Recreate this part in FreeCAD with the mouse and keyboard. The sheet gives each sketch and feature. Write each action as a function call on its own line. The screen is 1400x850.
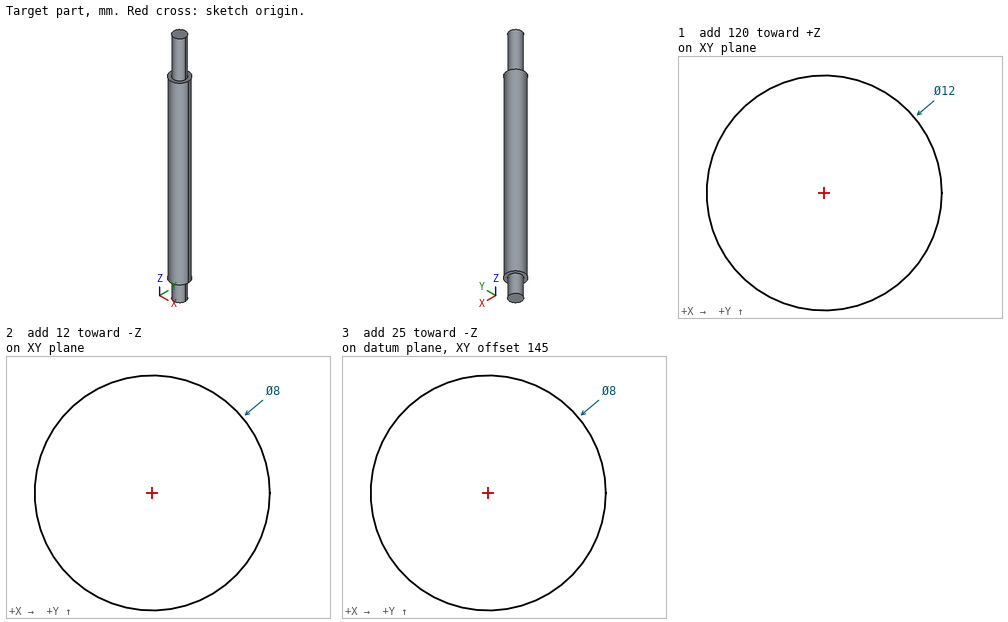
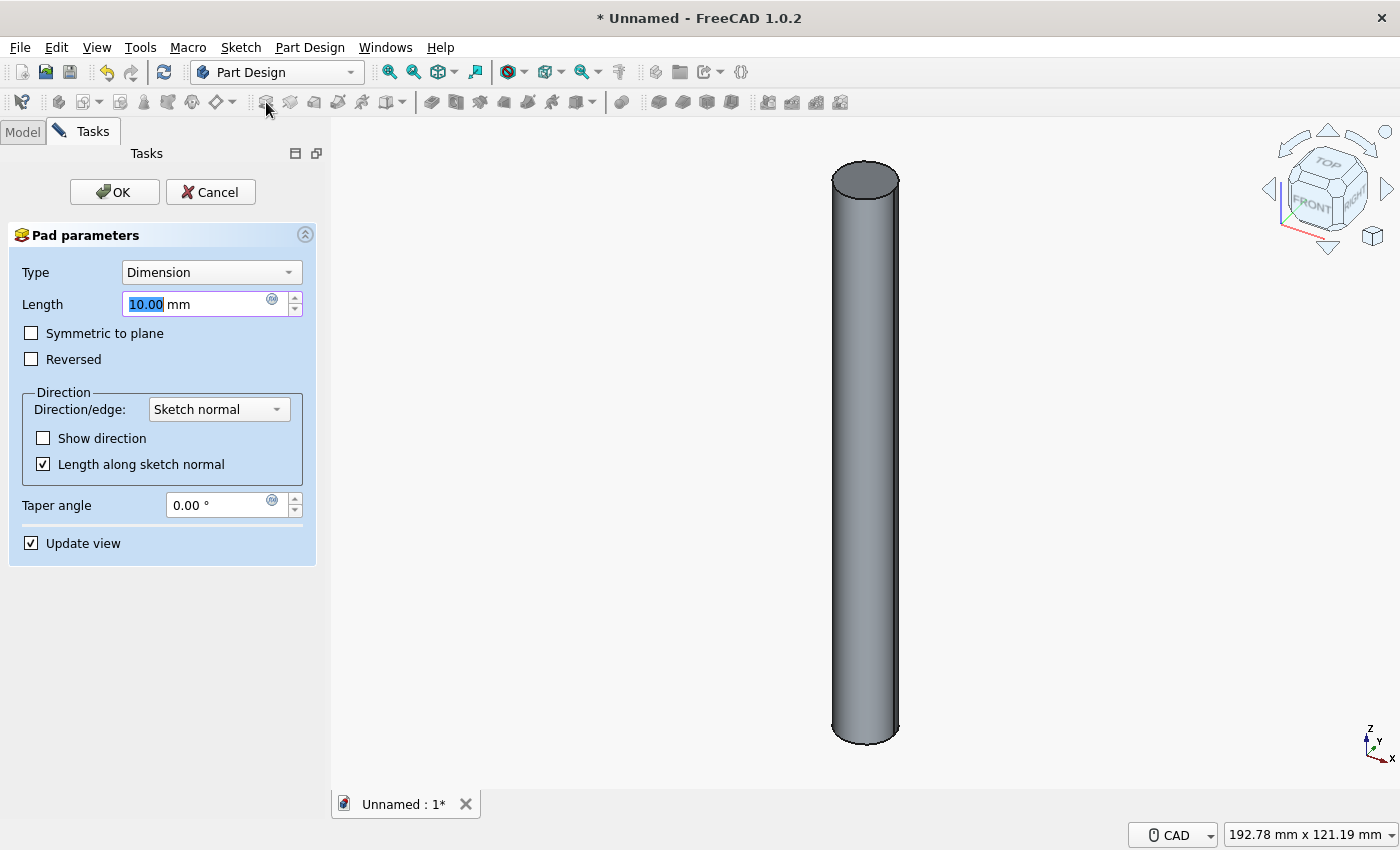
text(12)
key(Tab)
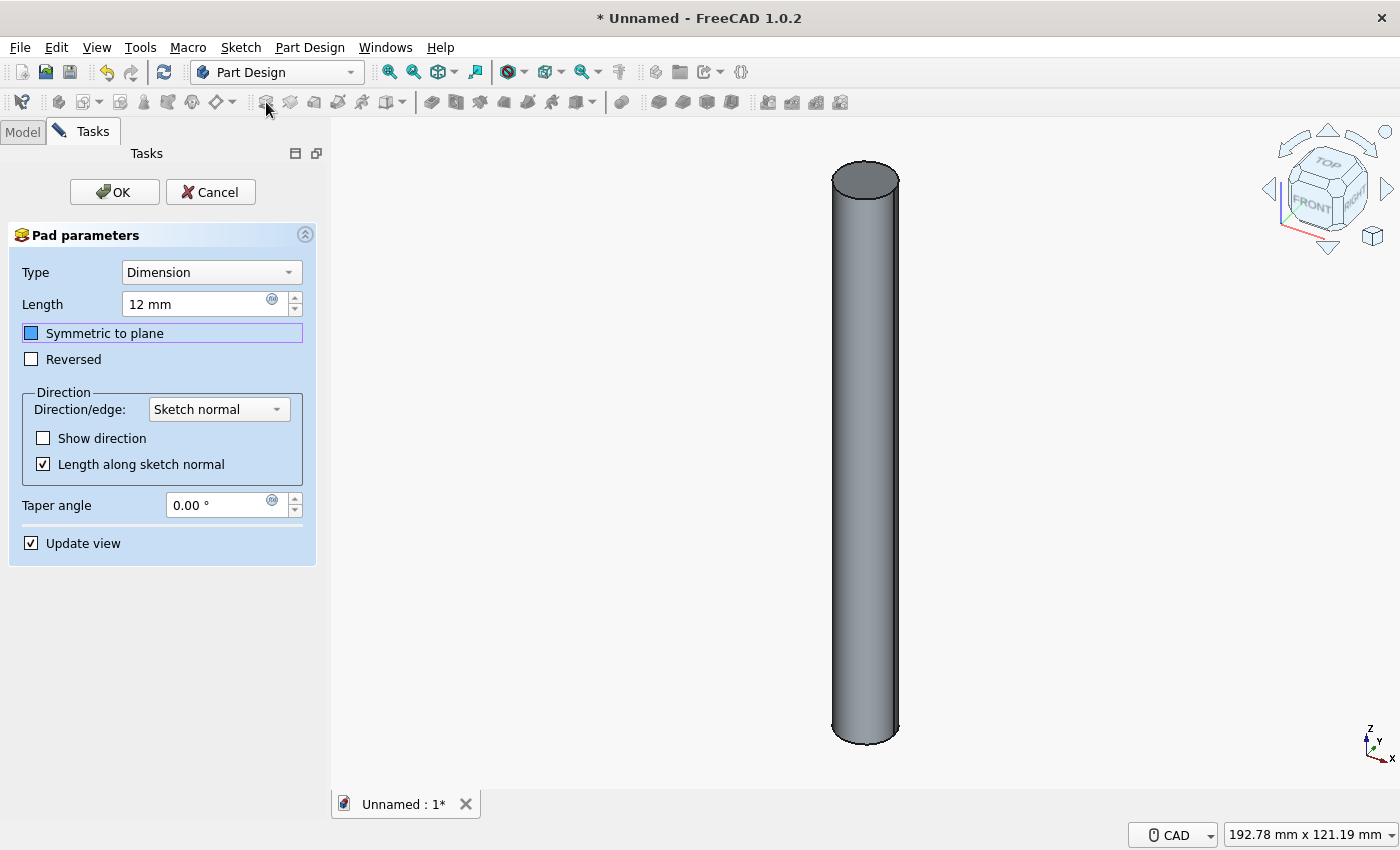
click(30, 359)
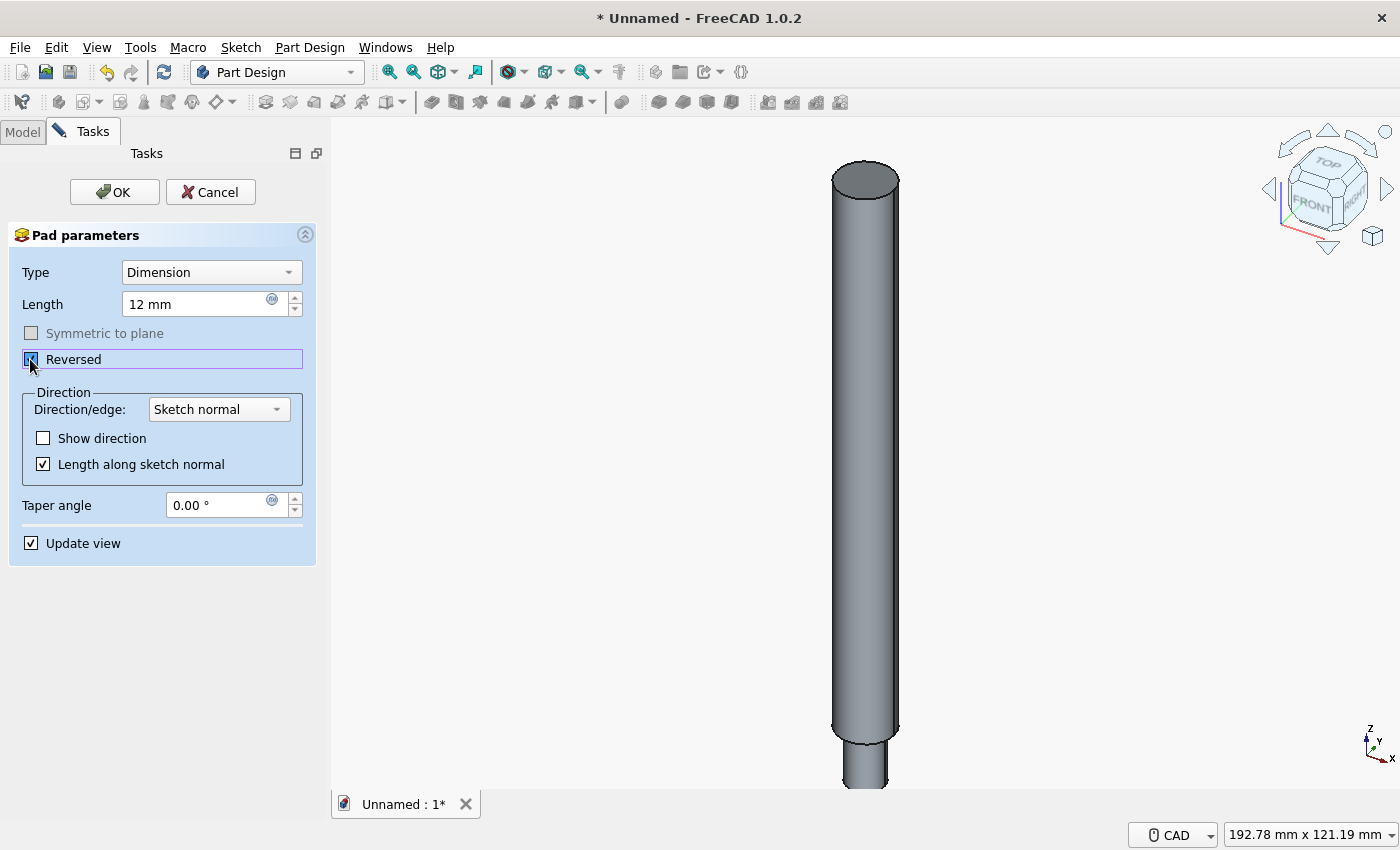
click(115, 192)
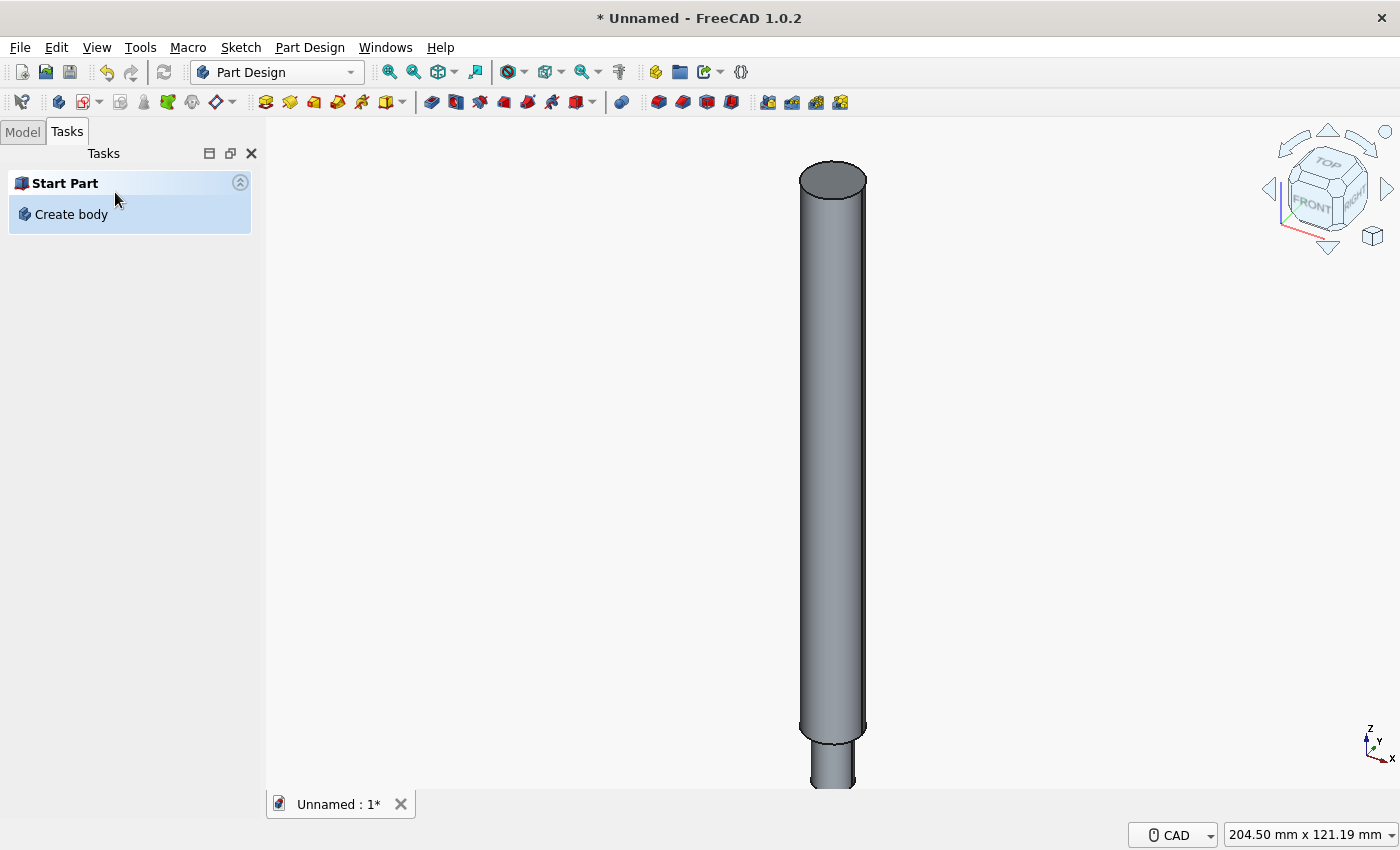
key(v)
key(f)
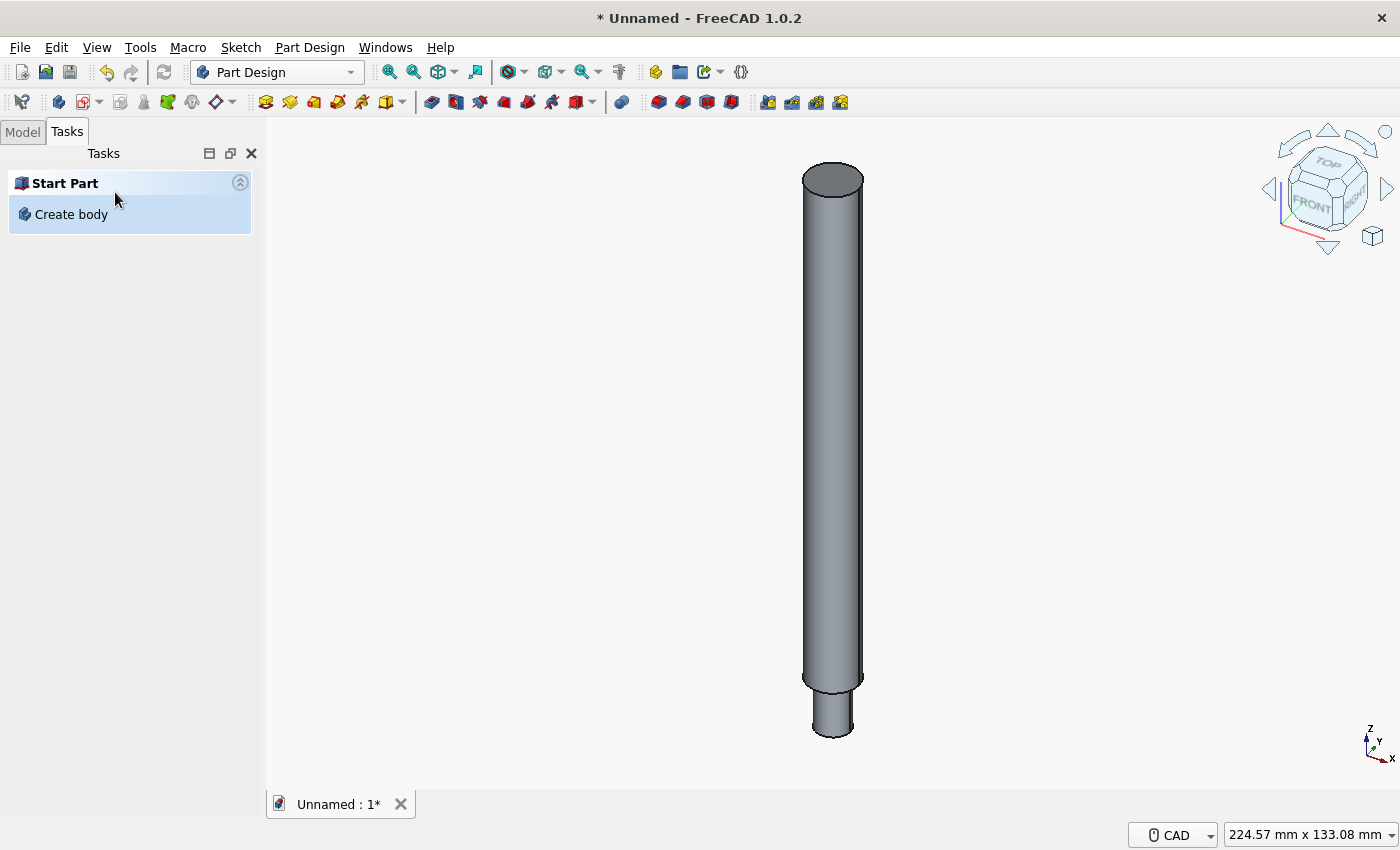
click(23, 131)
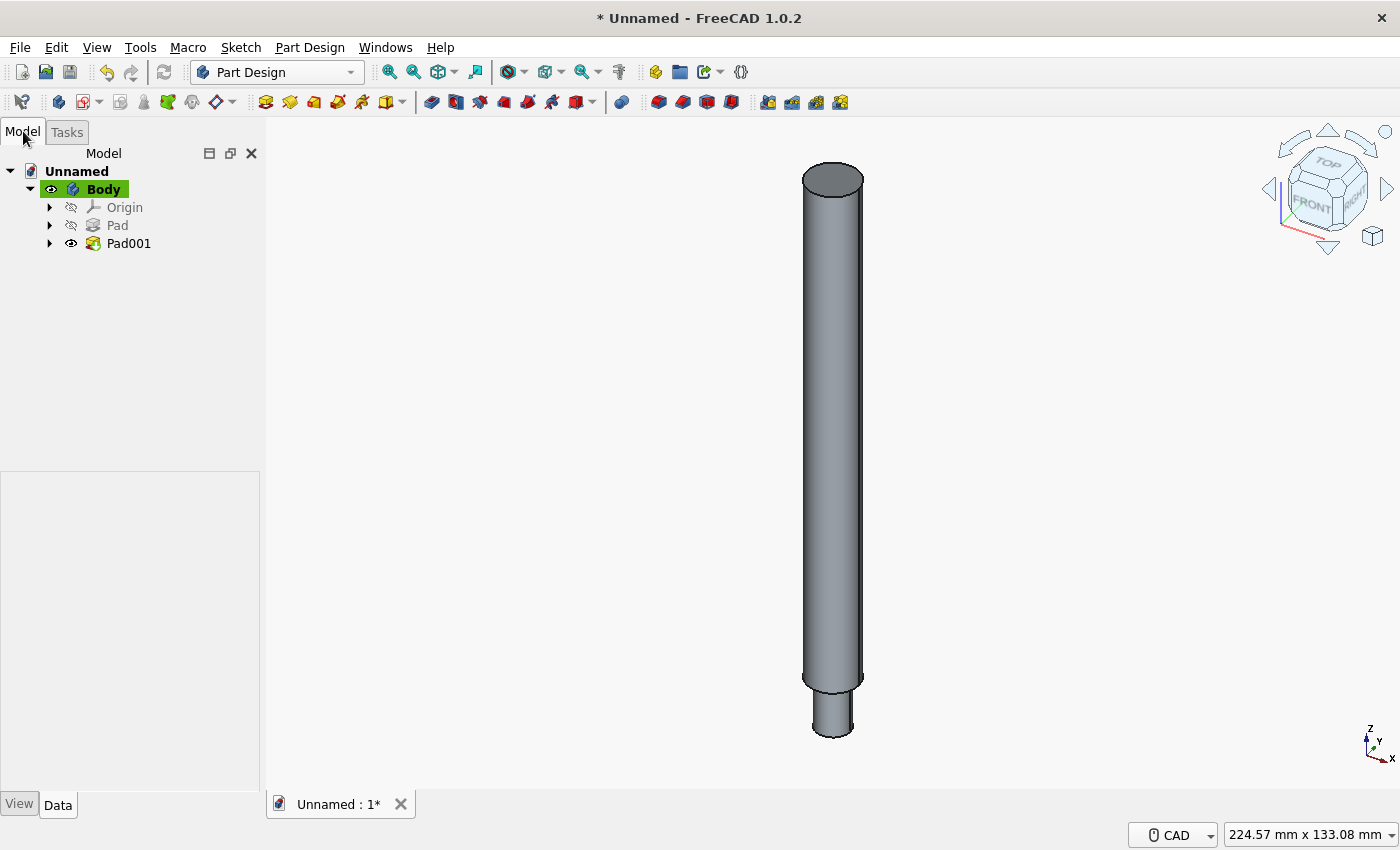
click(50, 207)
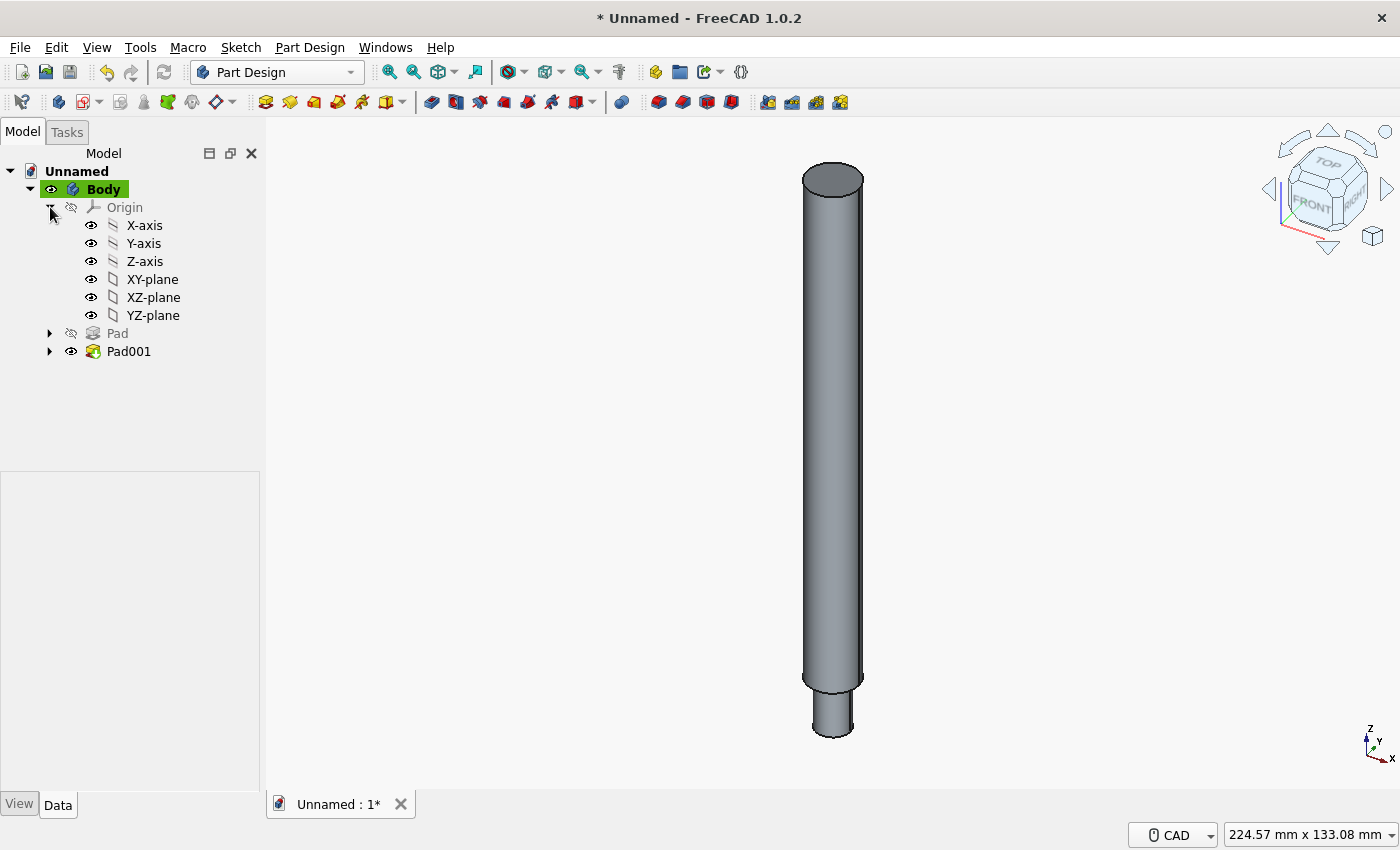
click(136, 279)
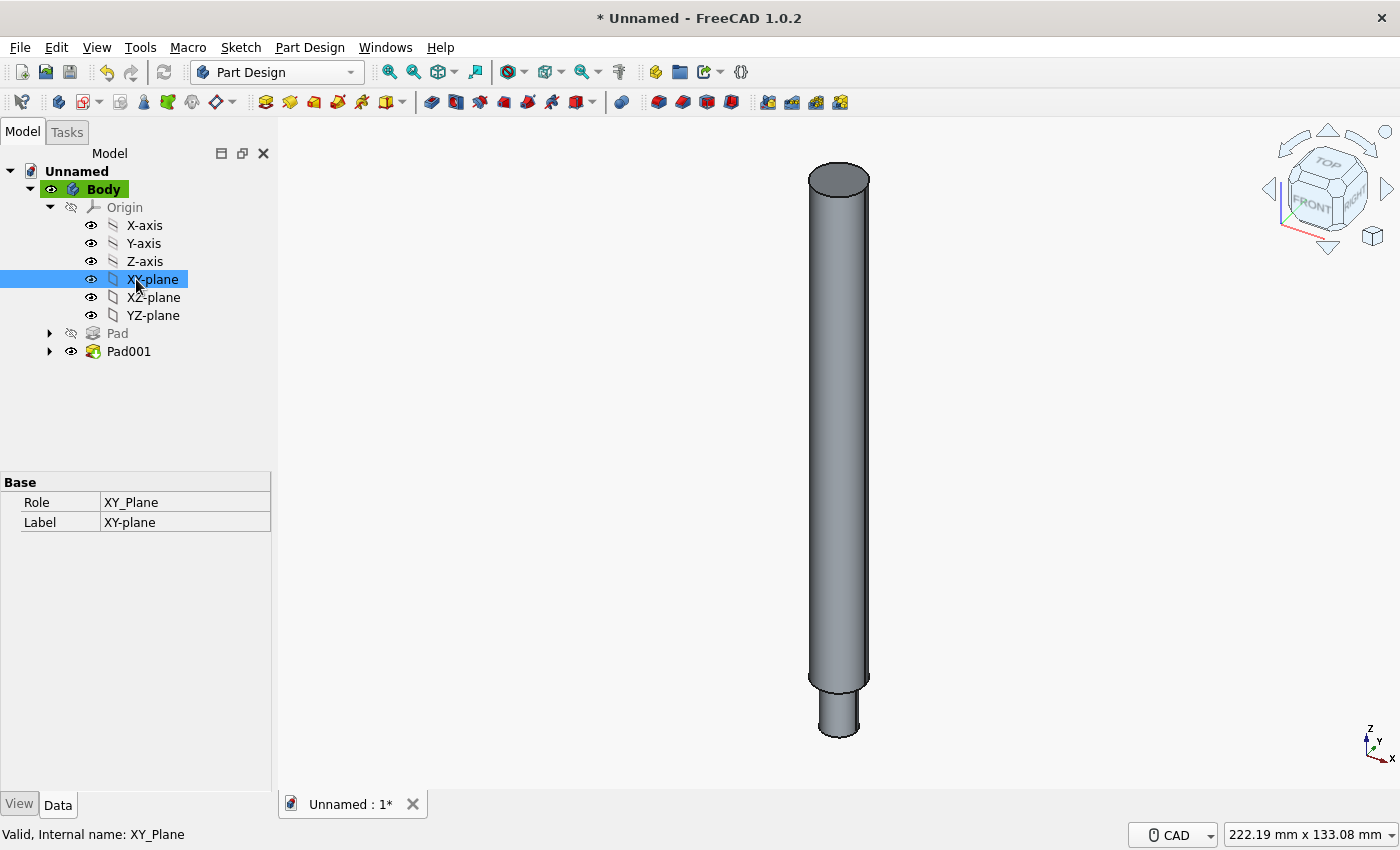
click(216, 102)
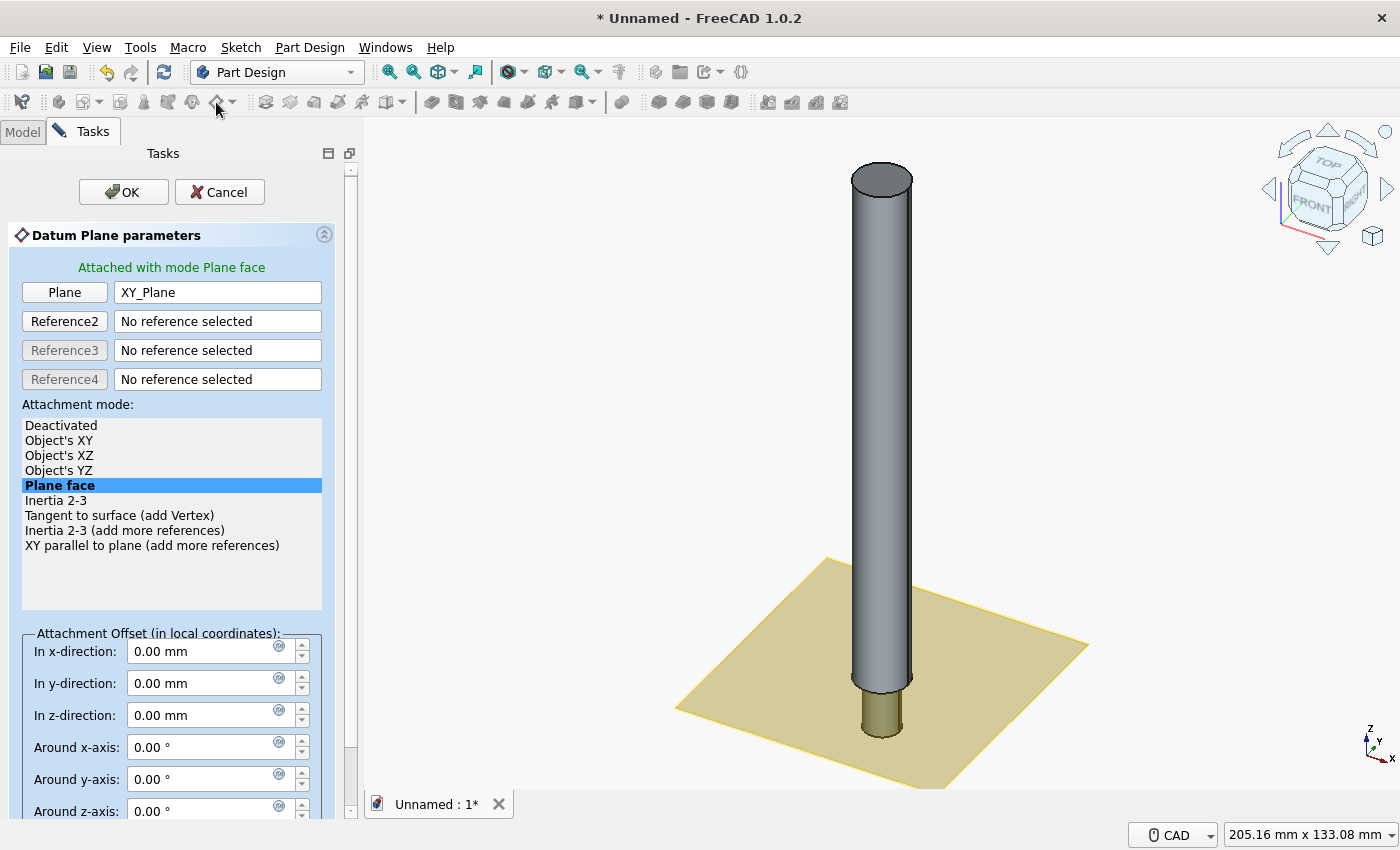
triple_click(210, 715)